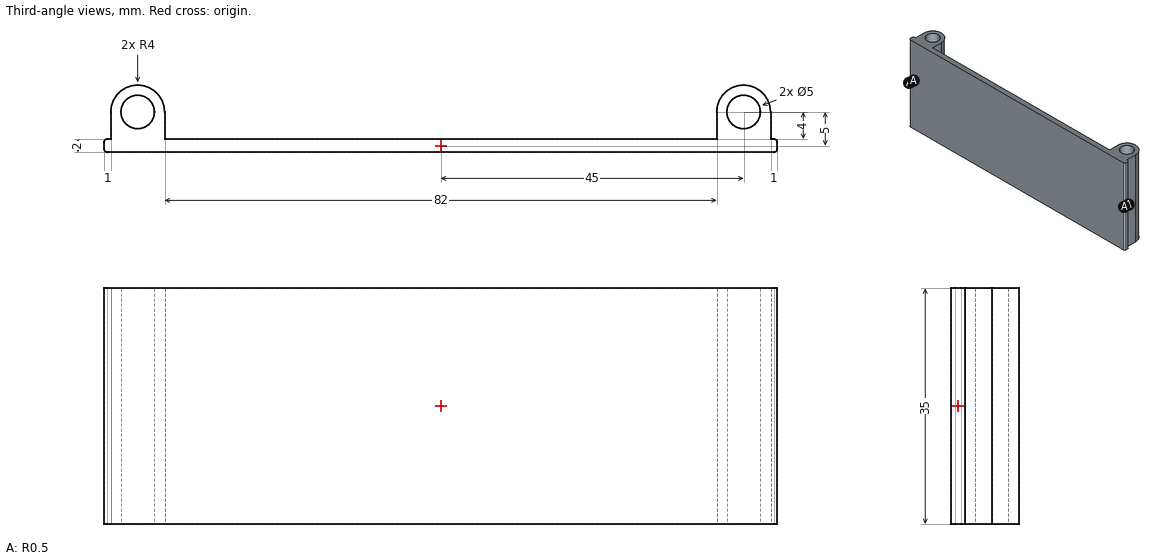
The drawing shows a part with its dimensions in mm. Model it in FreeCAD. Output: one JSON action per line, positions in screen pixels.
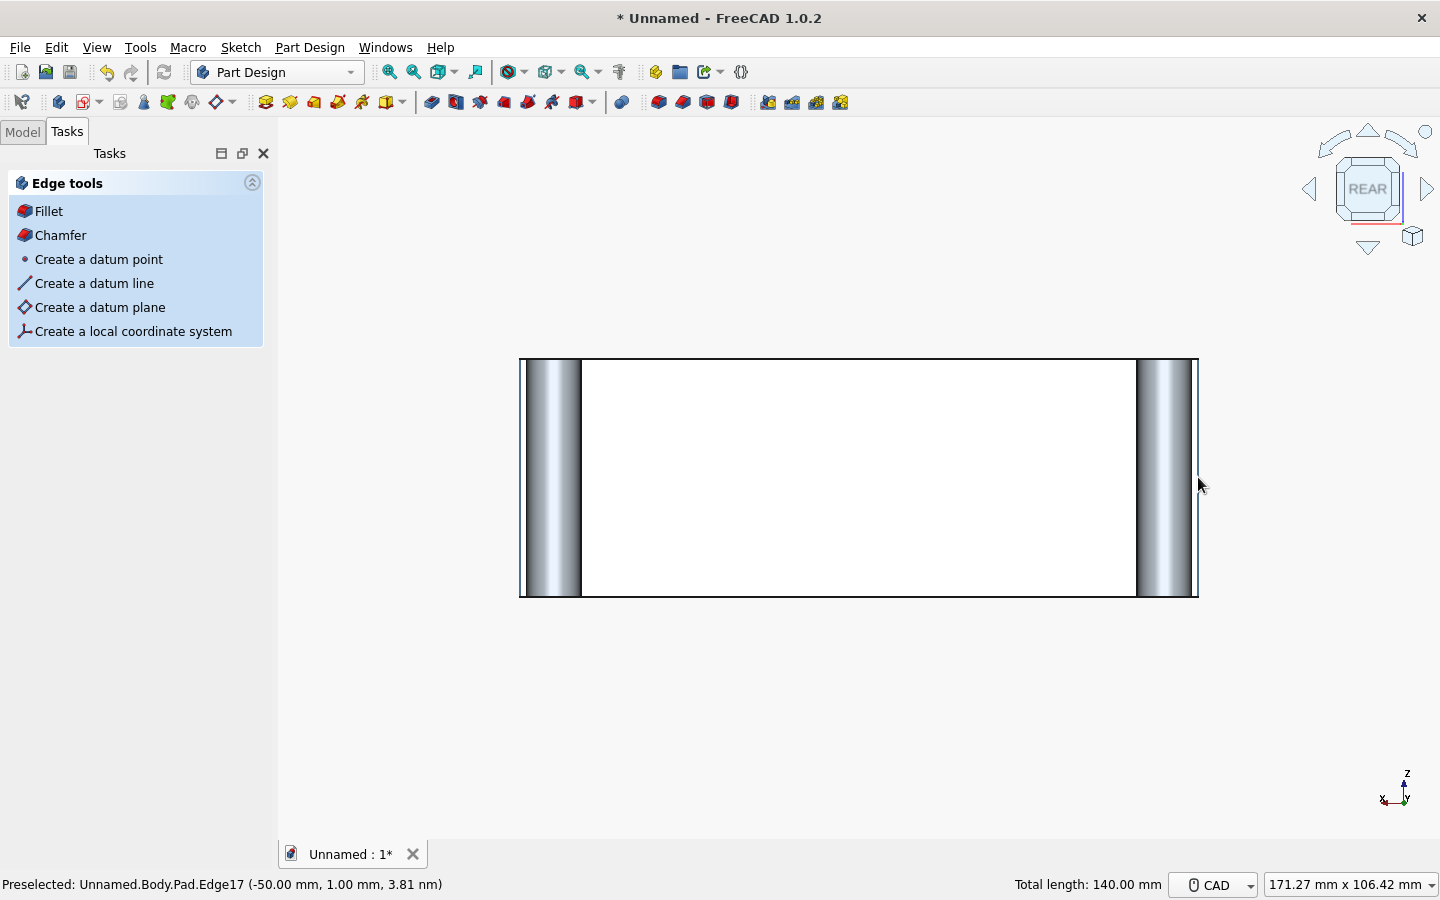
{"action": "left_click", "coordinate": [660, 102]}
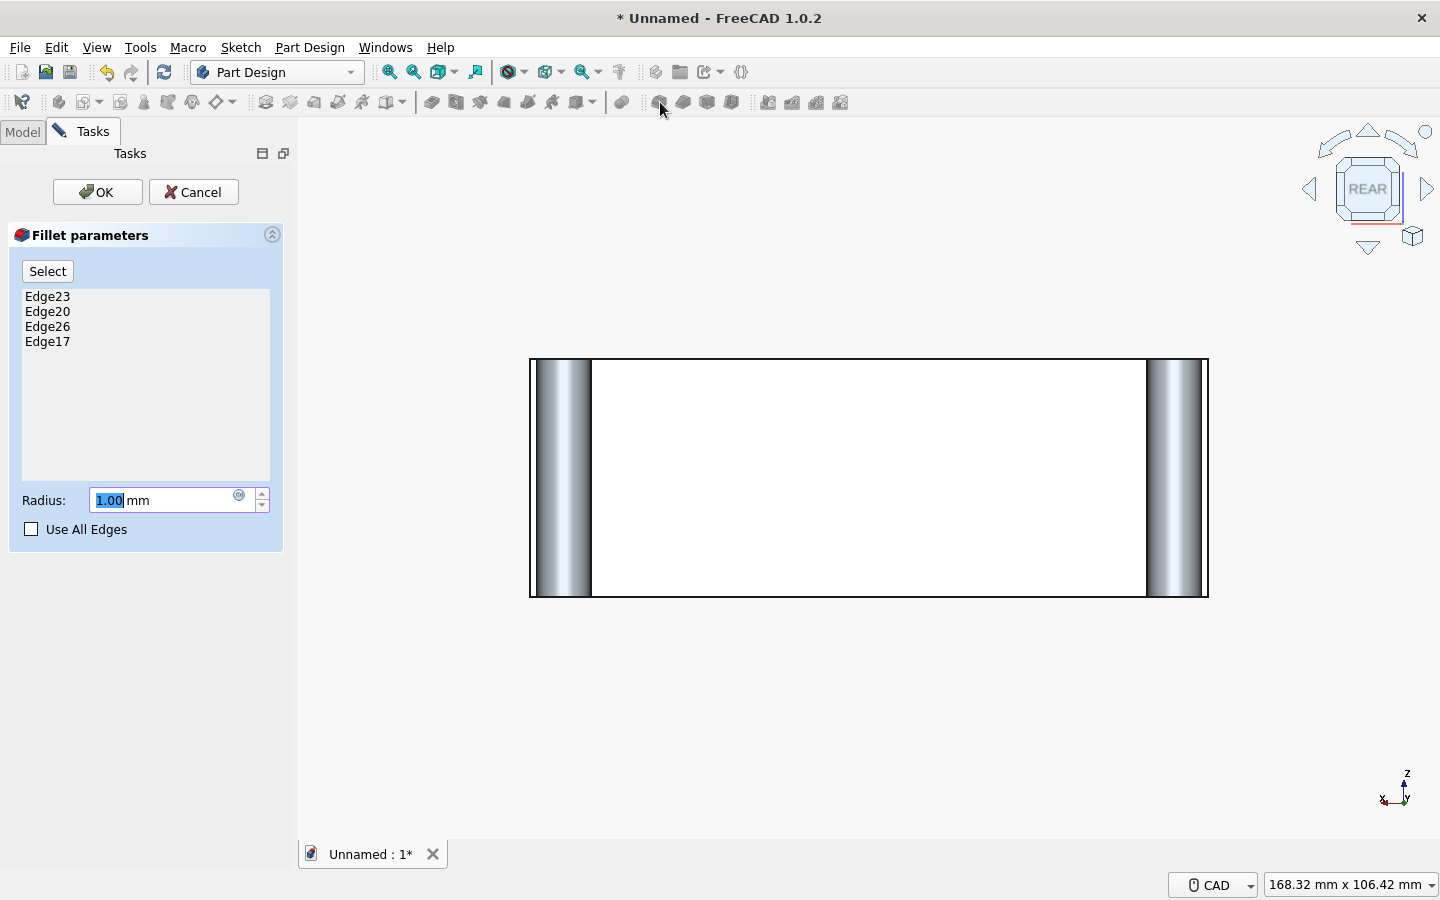
{"action": "type", "text": "0.5"}
{"action": "key", "text": "Tab"}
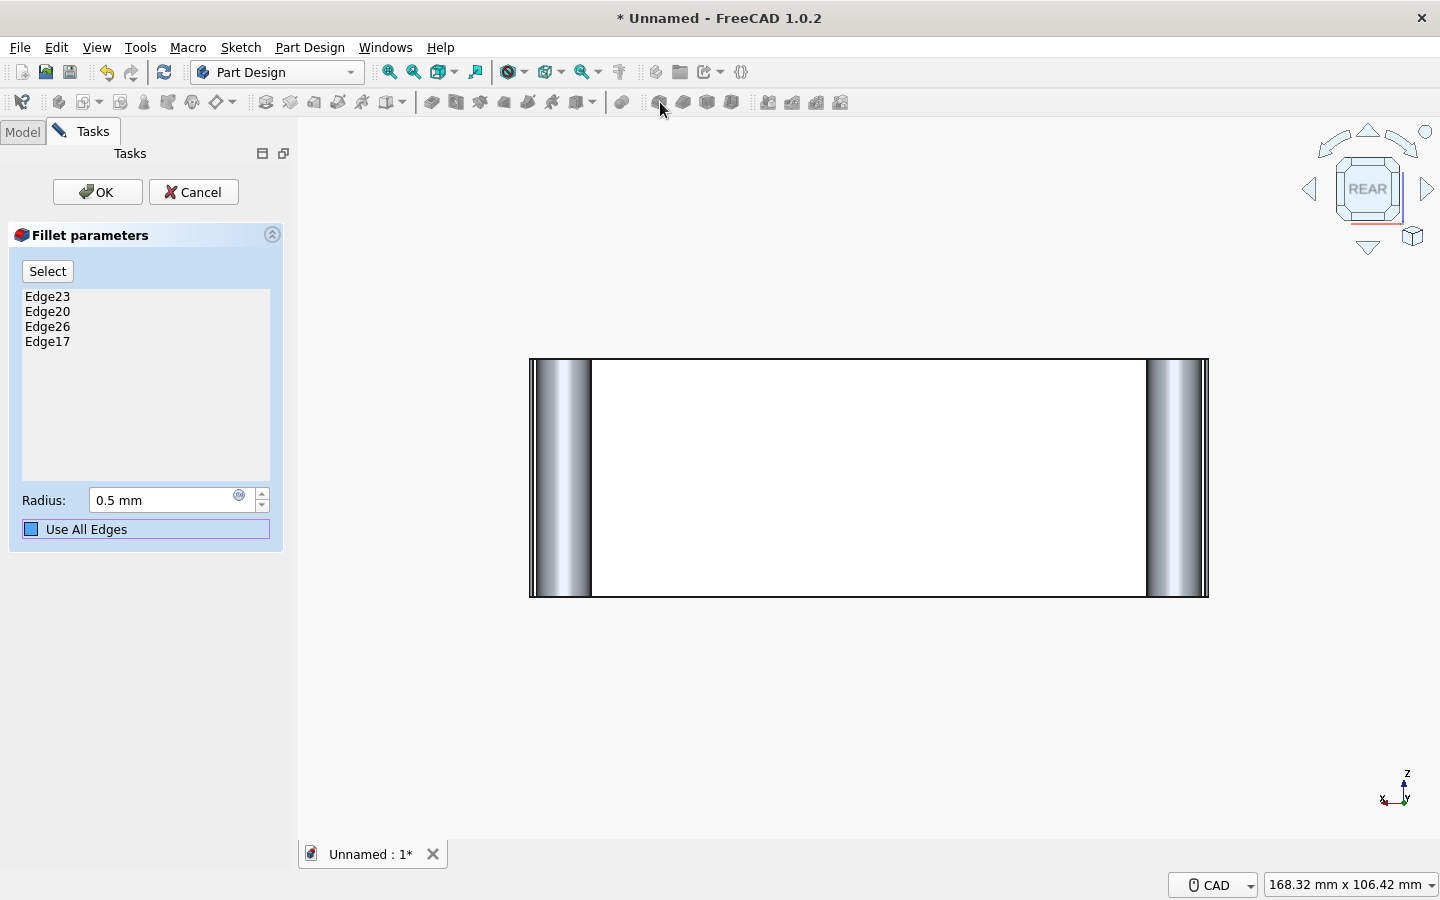
{"action": "left_click", "coordinate": [98, 192]}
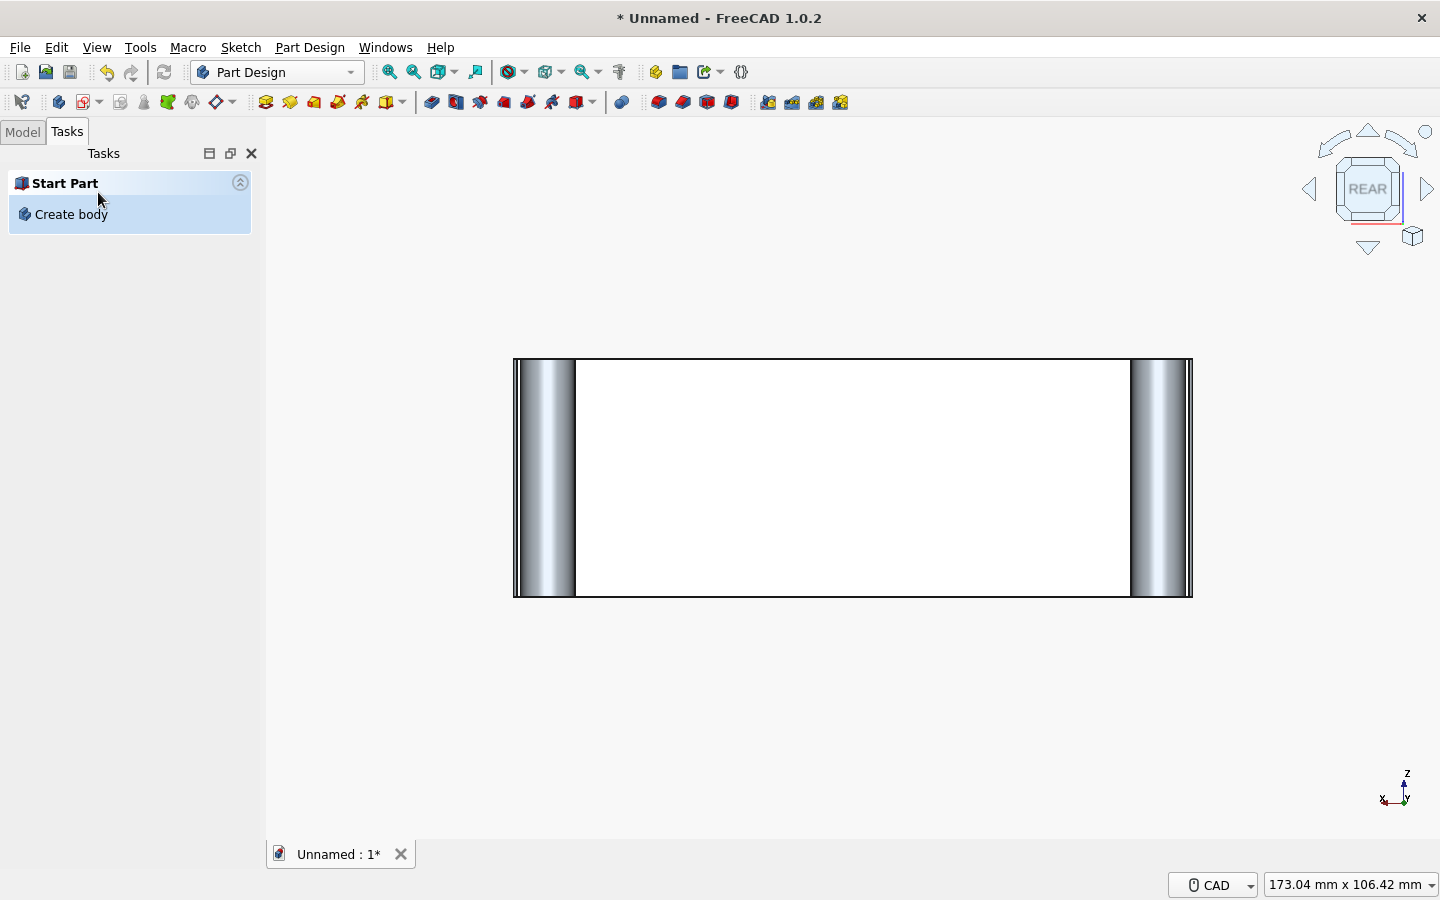
{"action": "key", "text": "0"}